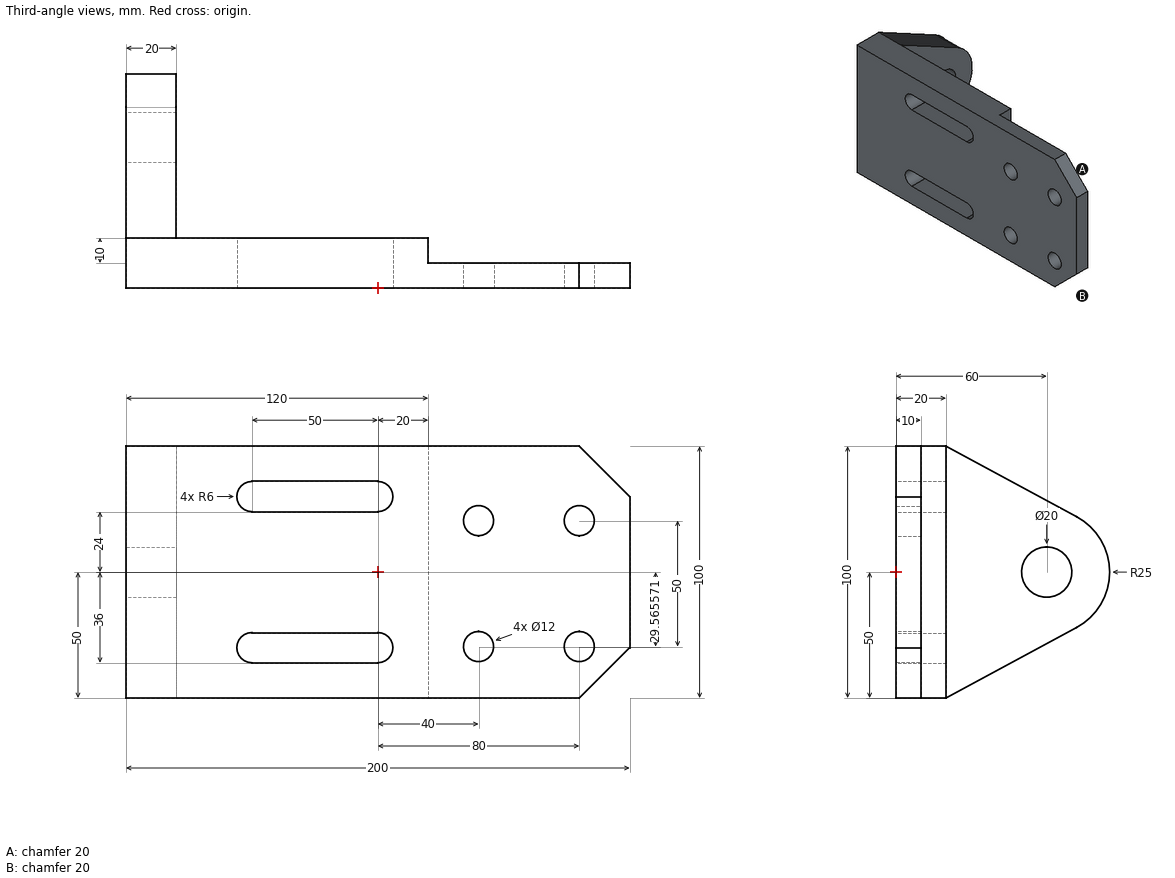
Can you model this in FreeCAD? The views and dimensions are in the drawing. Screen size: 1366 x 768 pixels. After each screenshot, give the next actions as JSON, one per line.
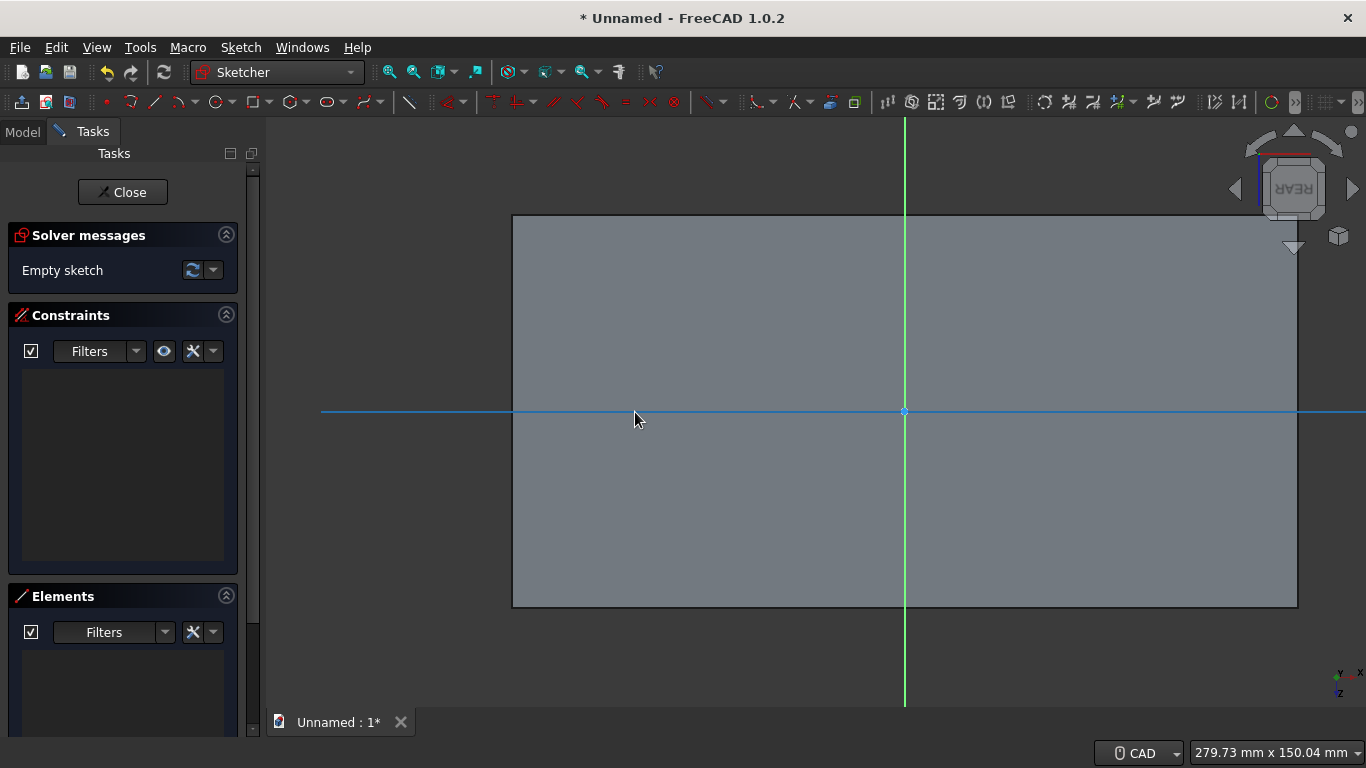
{"action": "left_click", "coordinate": [254, 102]}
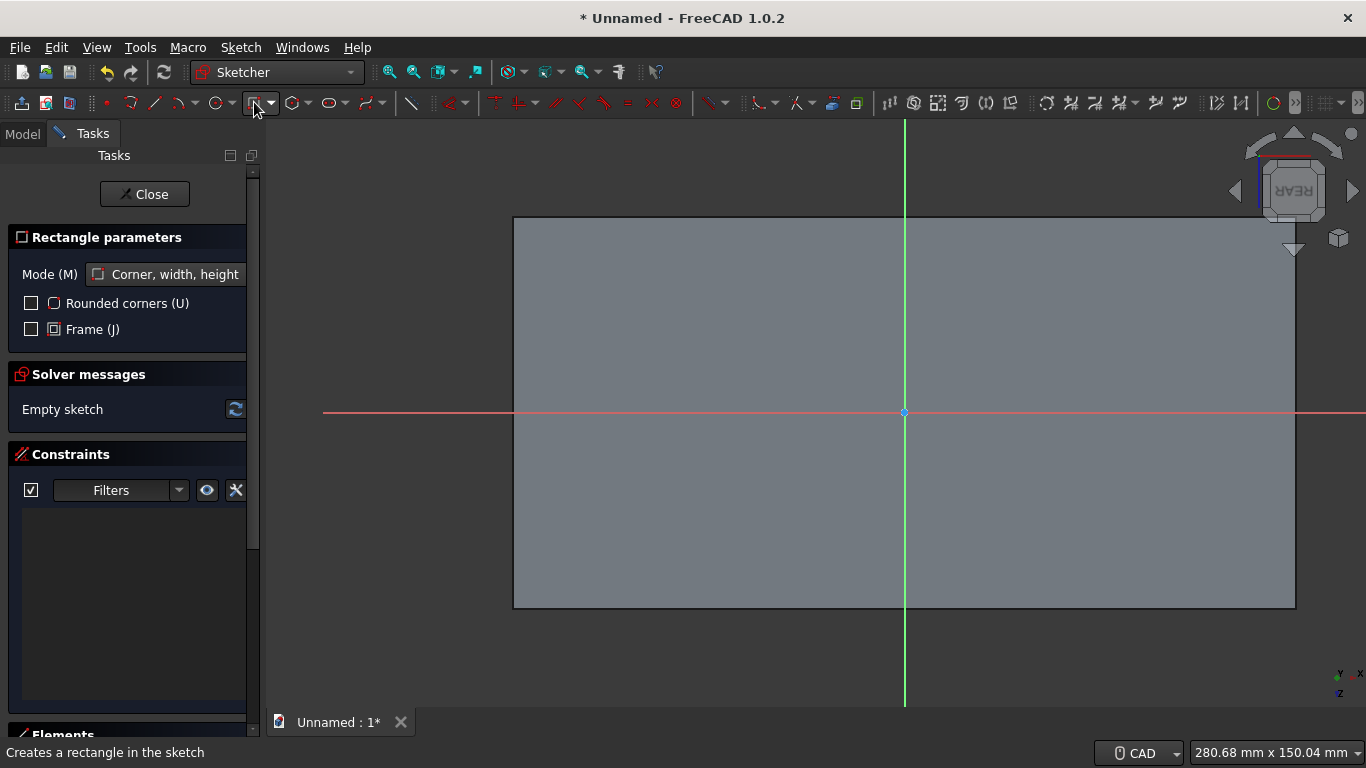
{"action": "left_click", "coordinate": [513, 217]}
{"action": "mouse_move", "coordinate": [983, 609]}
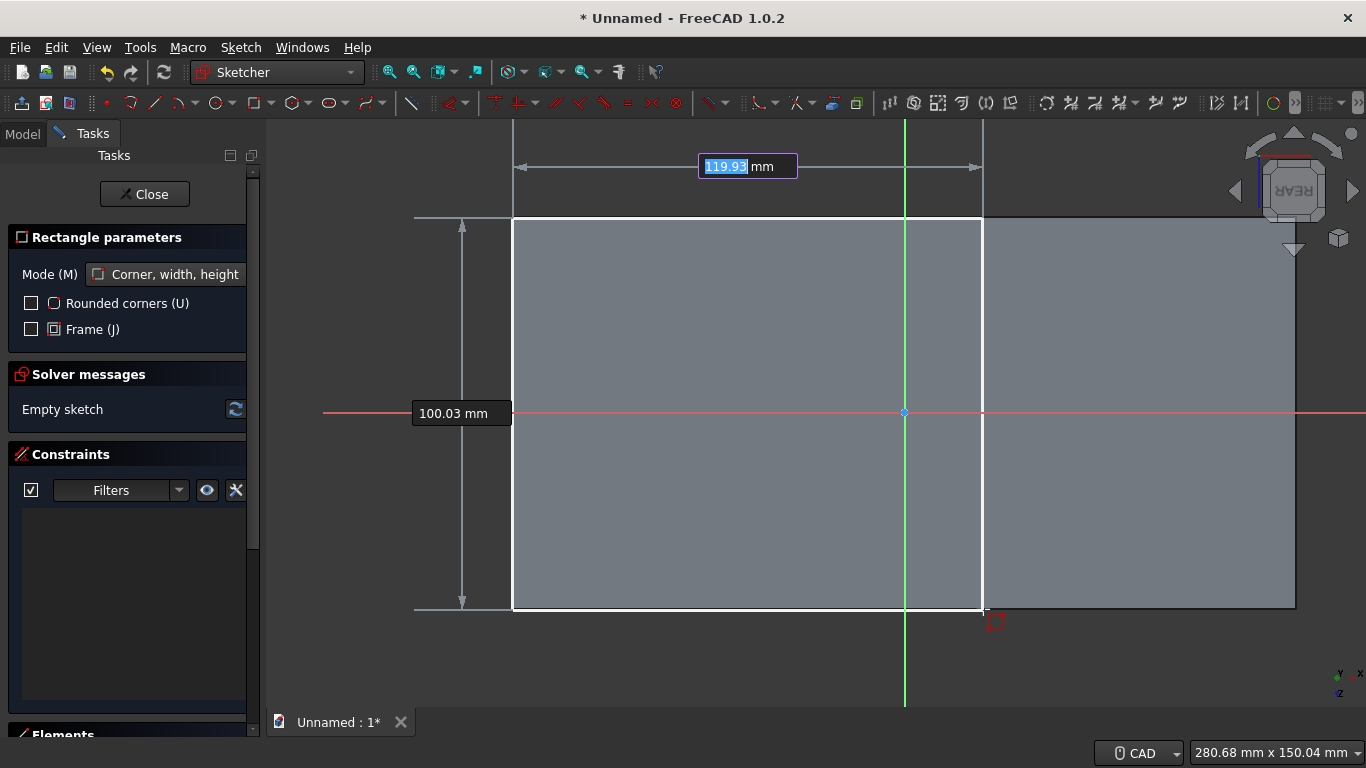
{"action": "type", "text": "120"}
{"action": "key", "text": "Tab"}
{"action": "type", "text": "100"}
{"action": "key", "text": "Return"}
{"action": "key", "text": "Escape"}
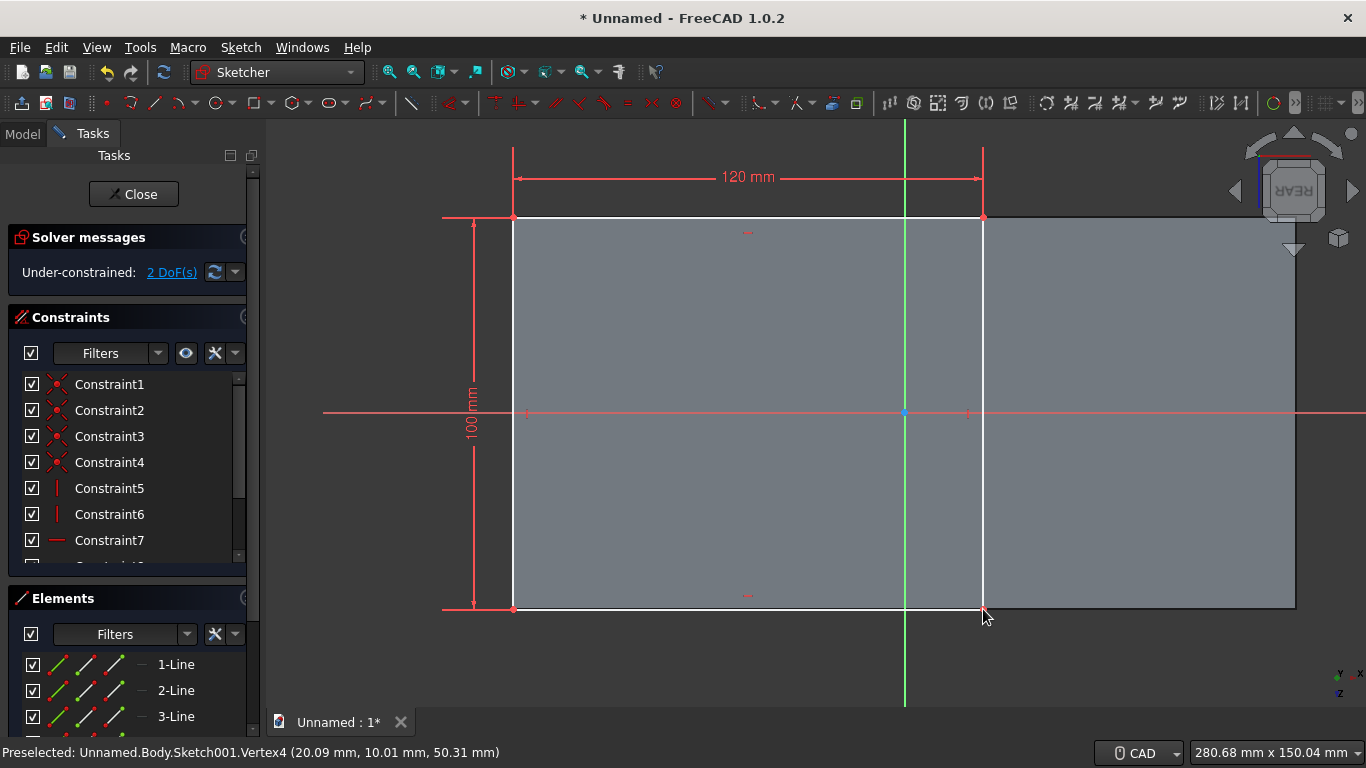
{"action": "left_click", "coordinate": [513, 218]}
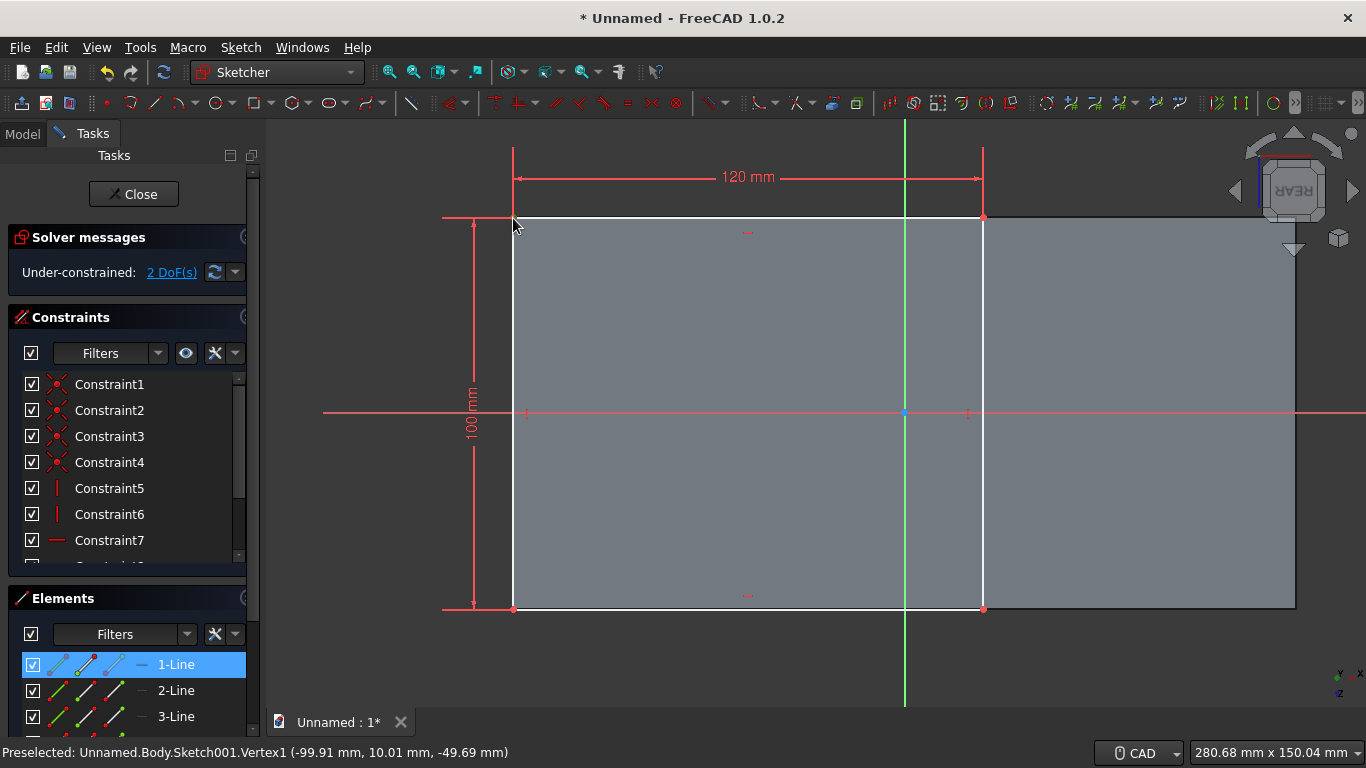
{"action": "key", "text": "i"}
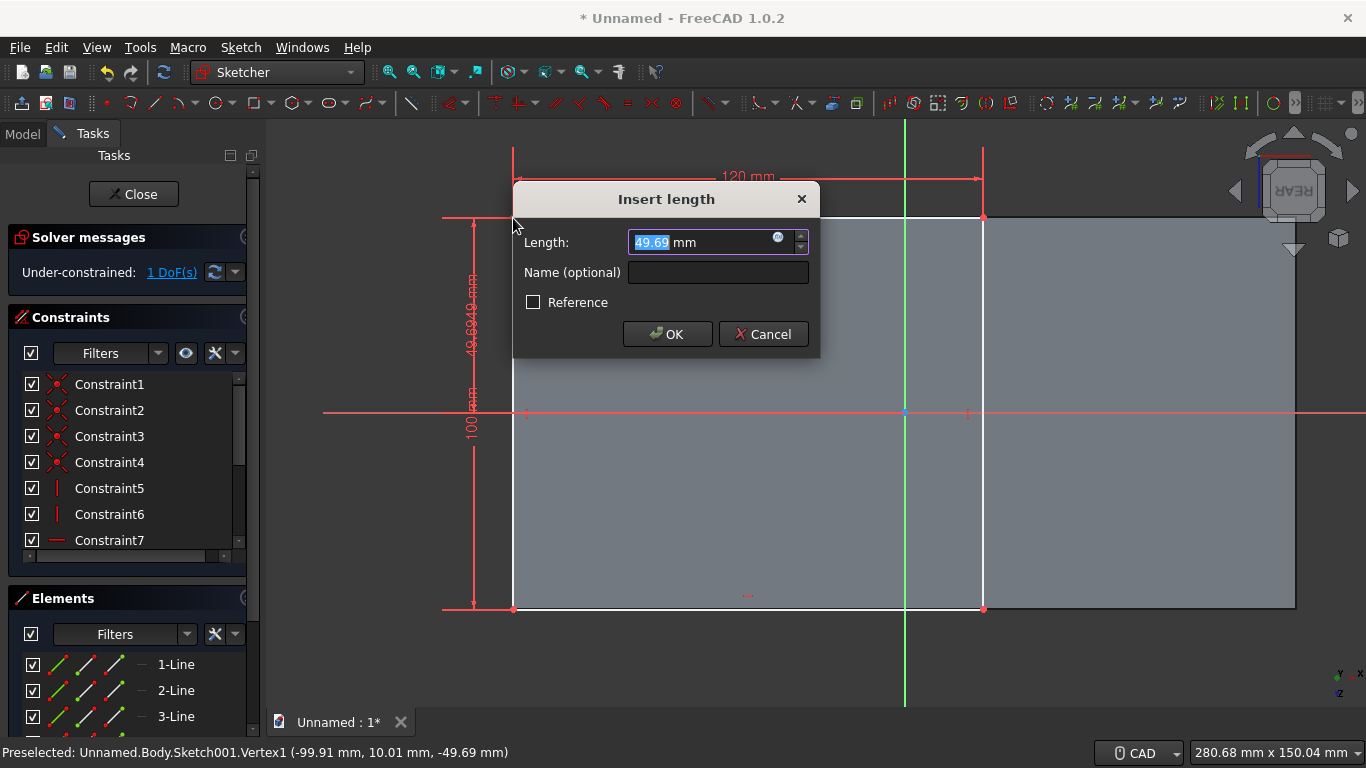
{"action": "type", "text": "50"}
{"action": "key", "text": "Return"}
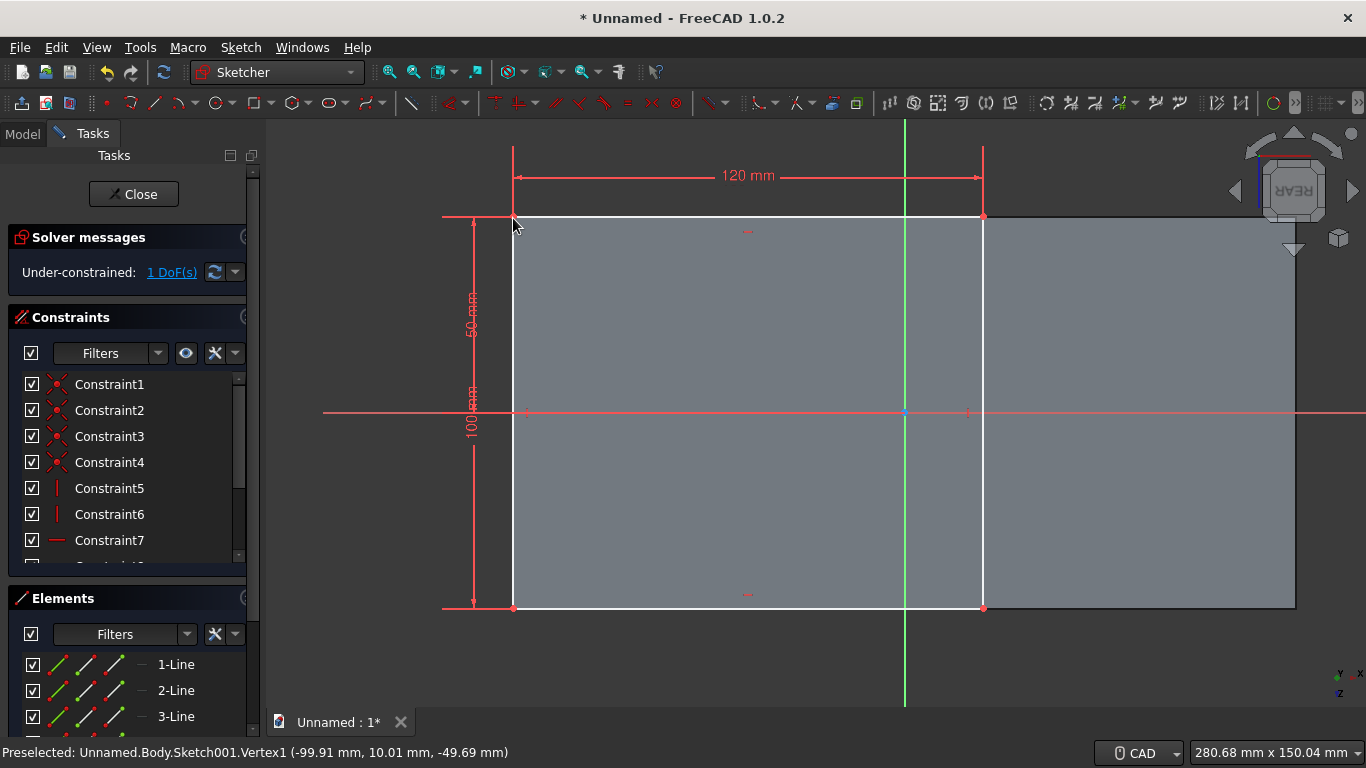
{"action": "left_click", "coordinate": [983, 609]}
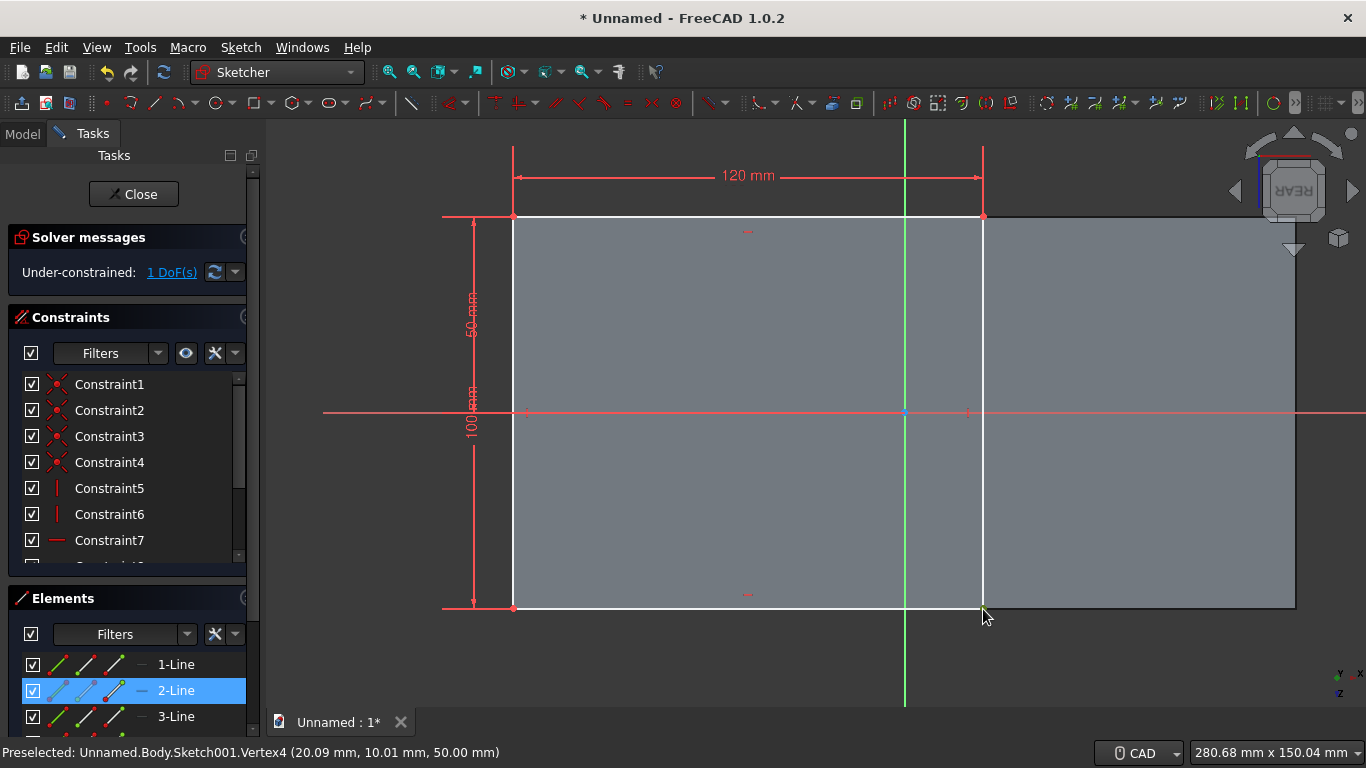
{"action": "left_click", "coordinate": [468, 104]}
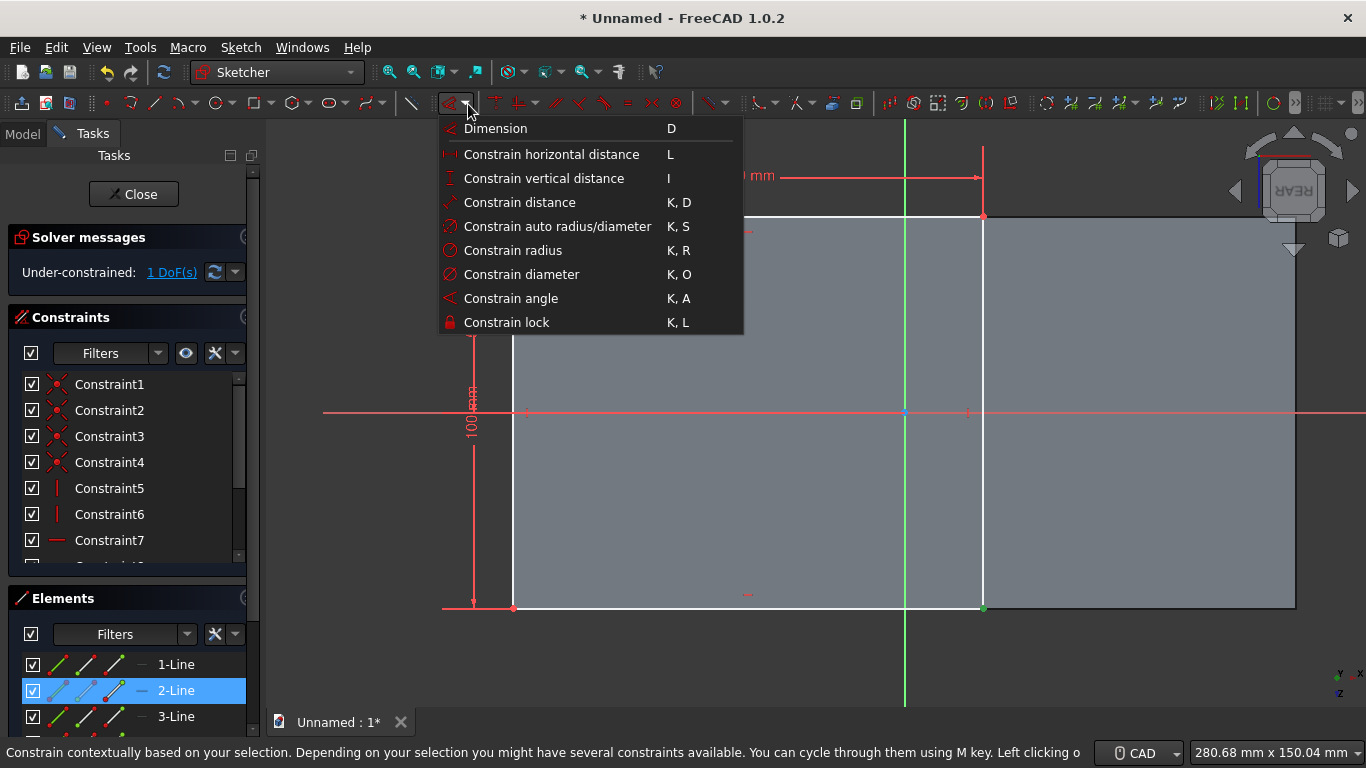
{"action": "left_click", "coordinate": [591, 154]}